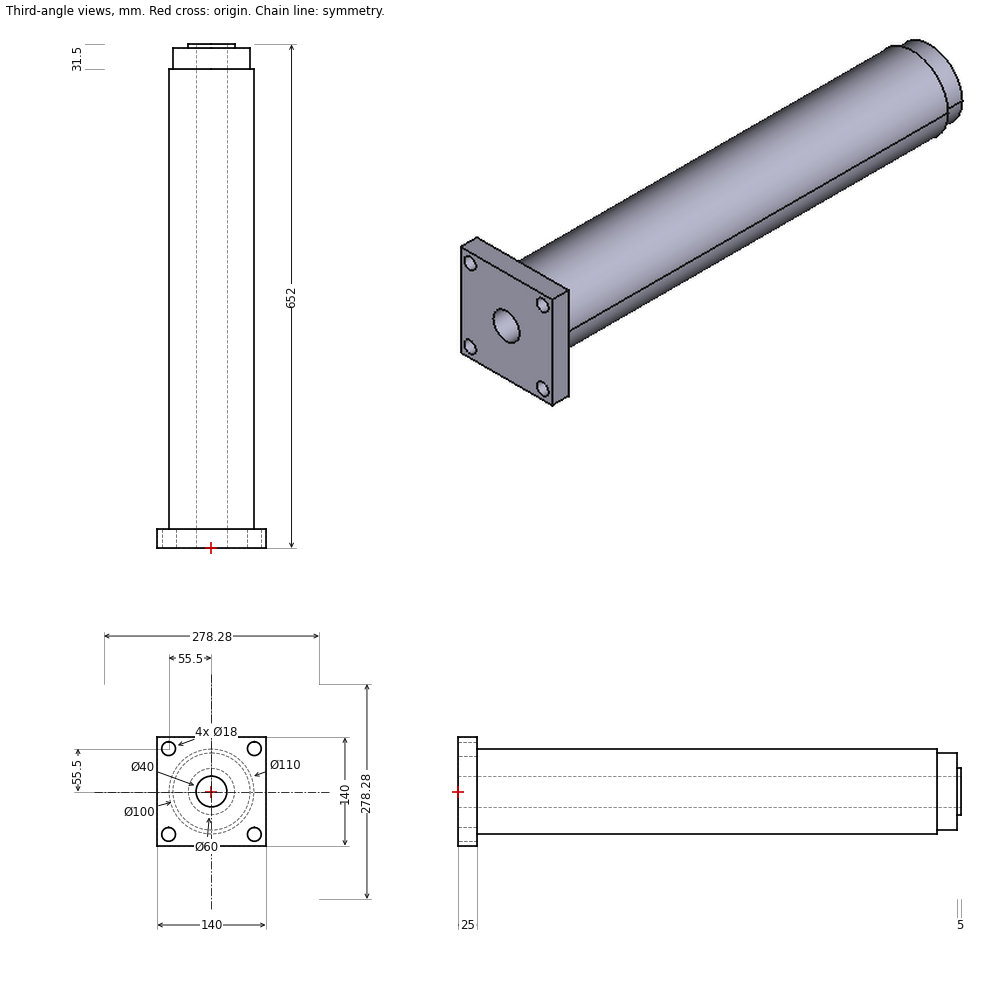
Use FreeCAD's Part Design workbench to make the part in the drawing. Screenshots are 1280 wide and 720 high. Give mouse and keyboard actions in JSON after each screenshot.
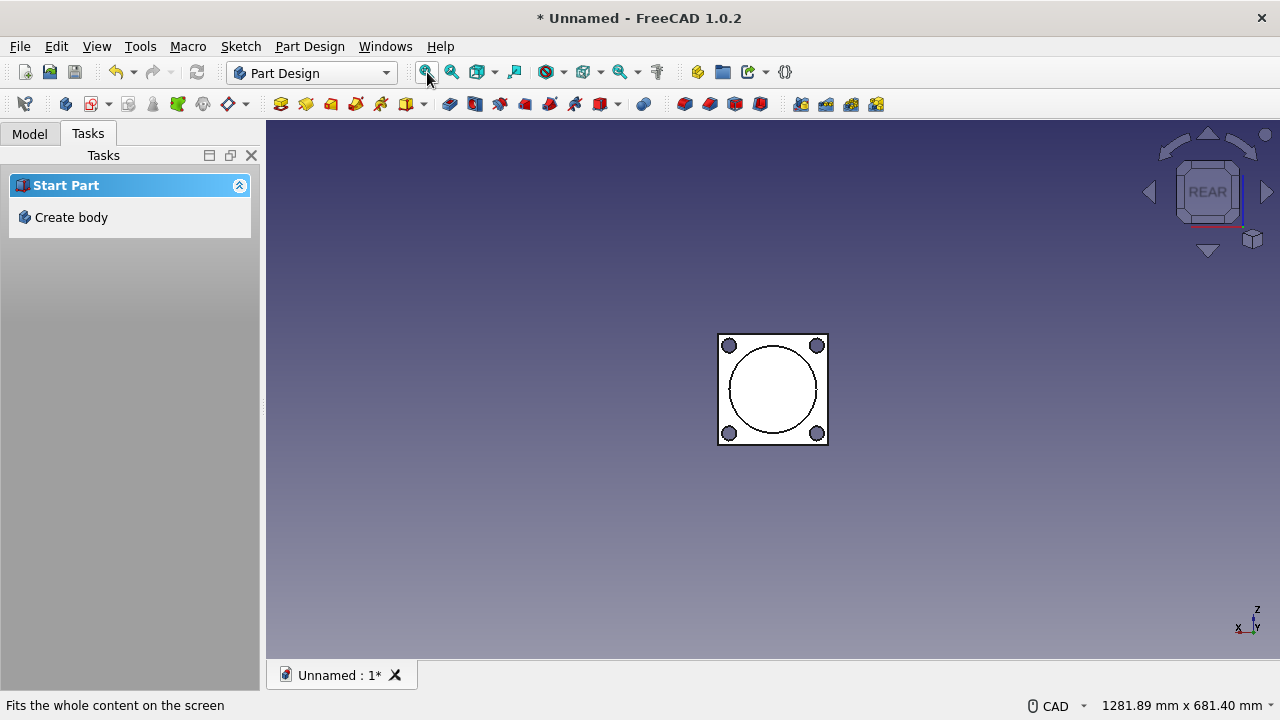
{"action": "left_click", "coordinate": [773, 389]}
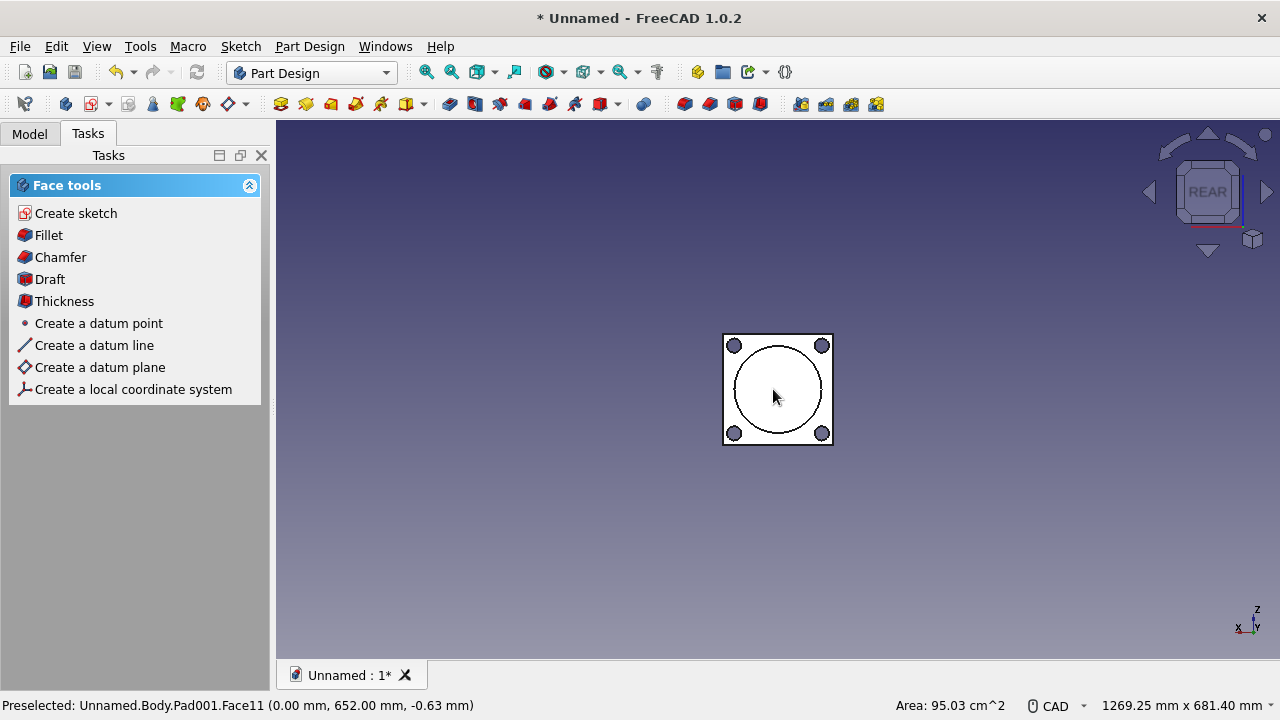
{"action": "left_click", "coordinate": [90, 104]}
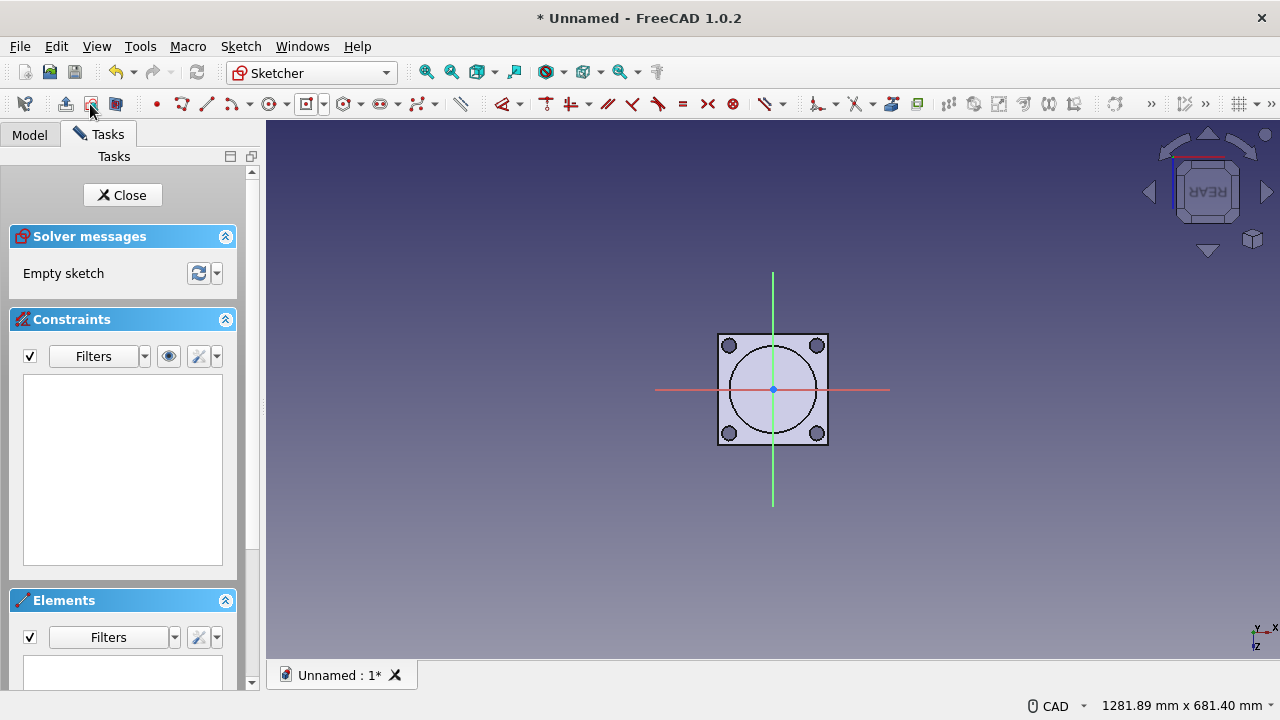
{"action": "scroll", "coordinate": [780, 389], "scroll_direction": "up", "scroll_amount": 12}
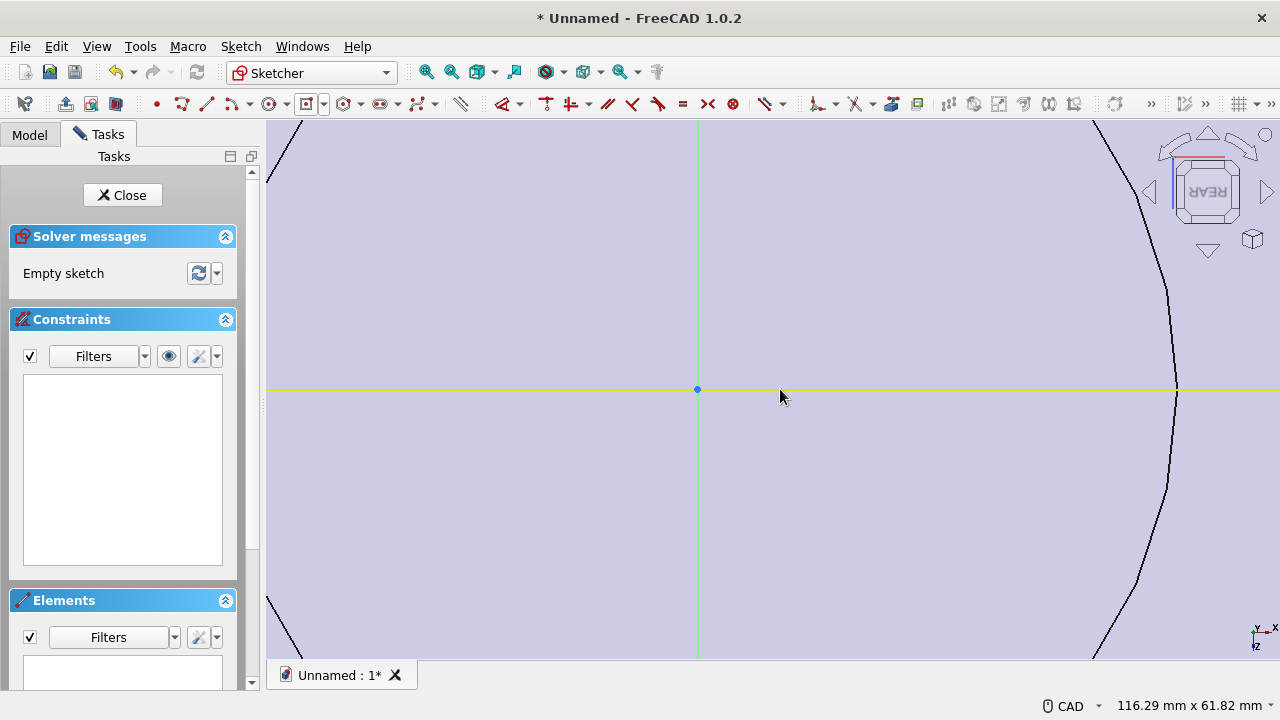
{"action": "key", "text": "g c"}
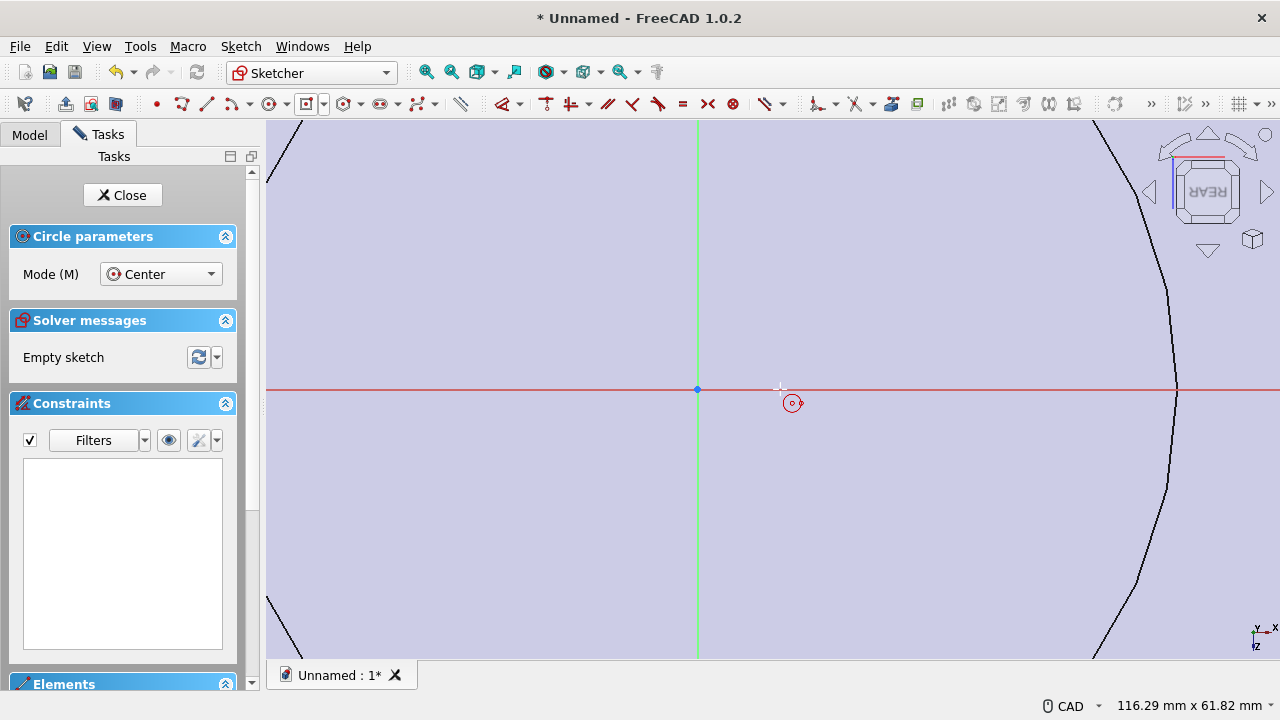
{"action": "left_click", "coordinate": [698, 389]}
{"action": "mouse_move", "coordinate": [821, 266]}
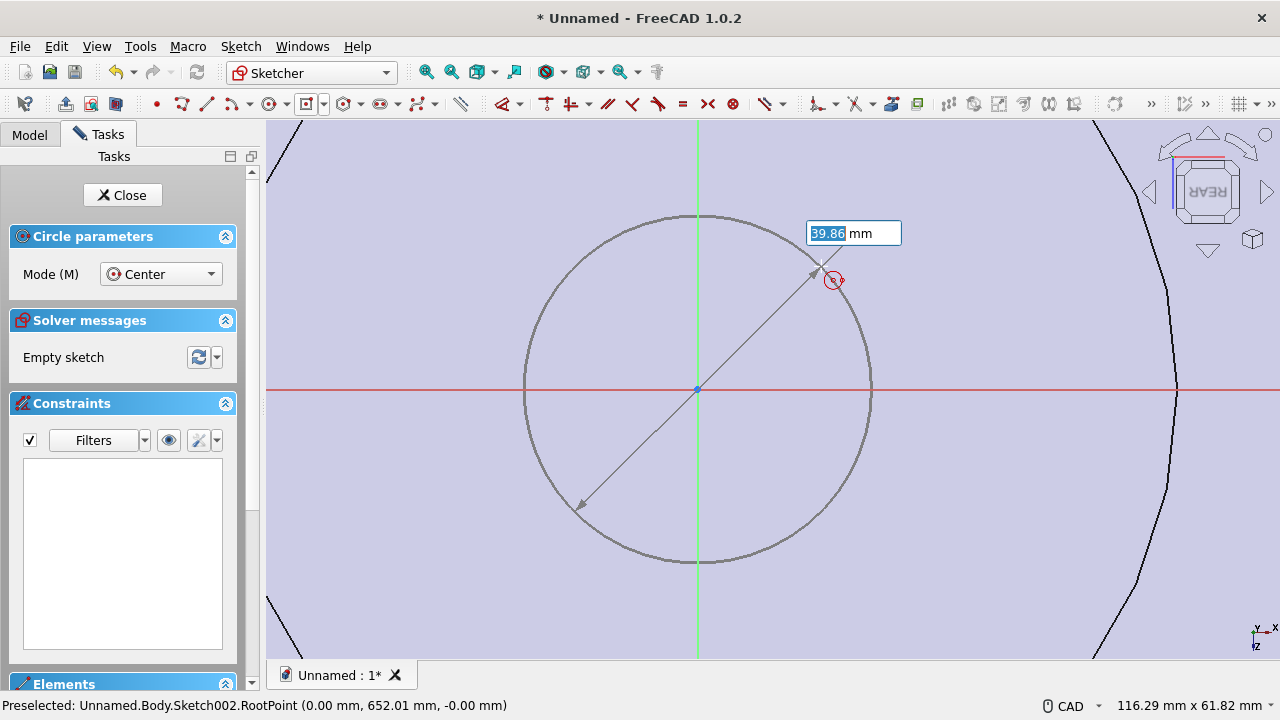
{"action": "type", "text": "40"}
{"action": "key", "text": "Return"}
{"action": "key", "text": "Escape"}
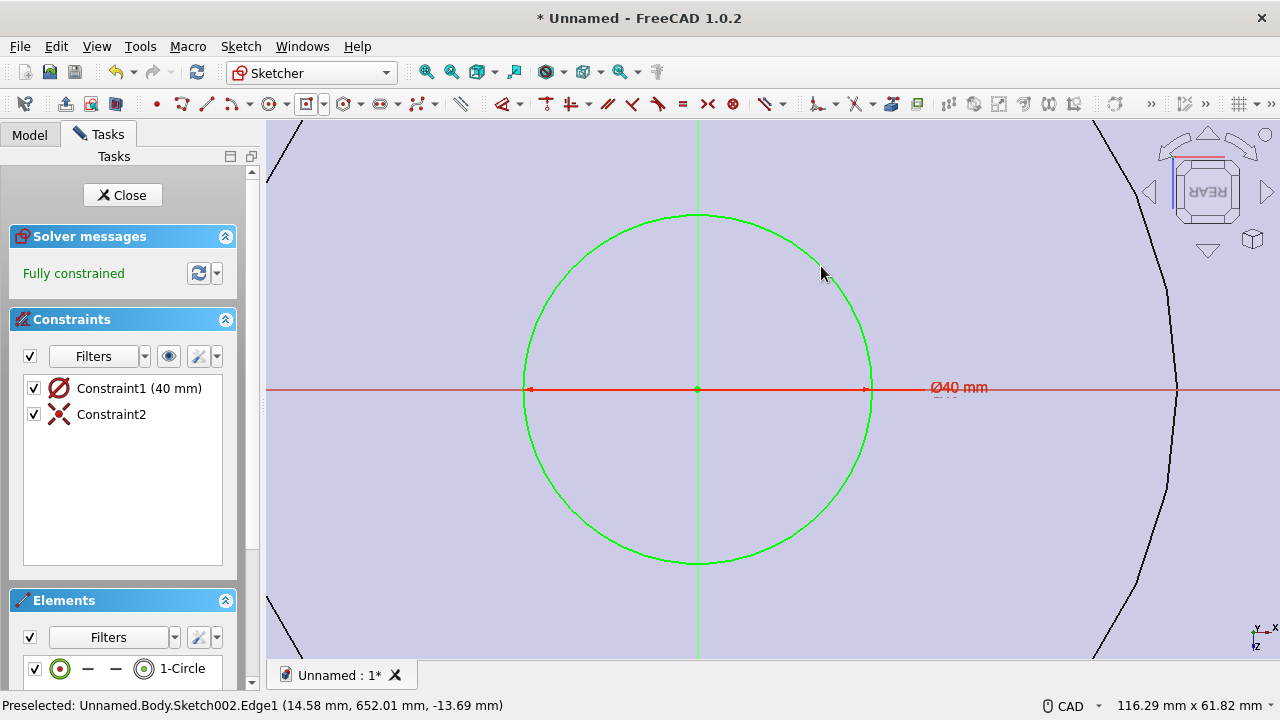
{"action": "left_click", "coordinate": [123, 195]}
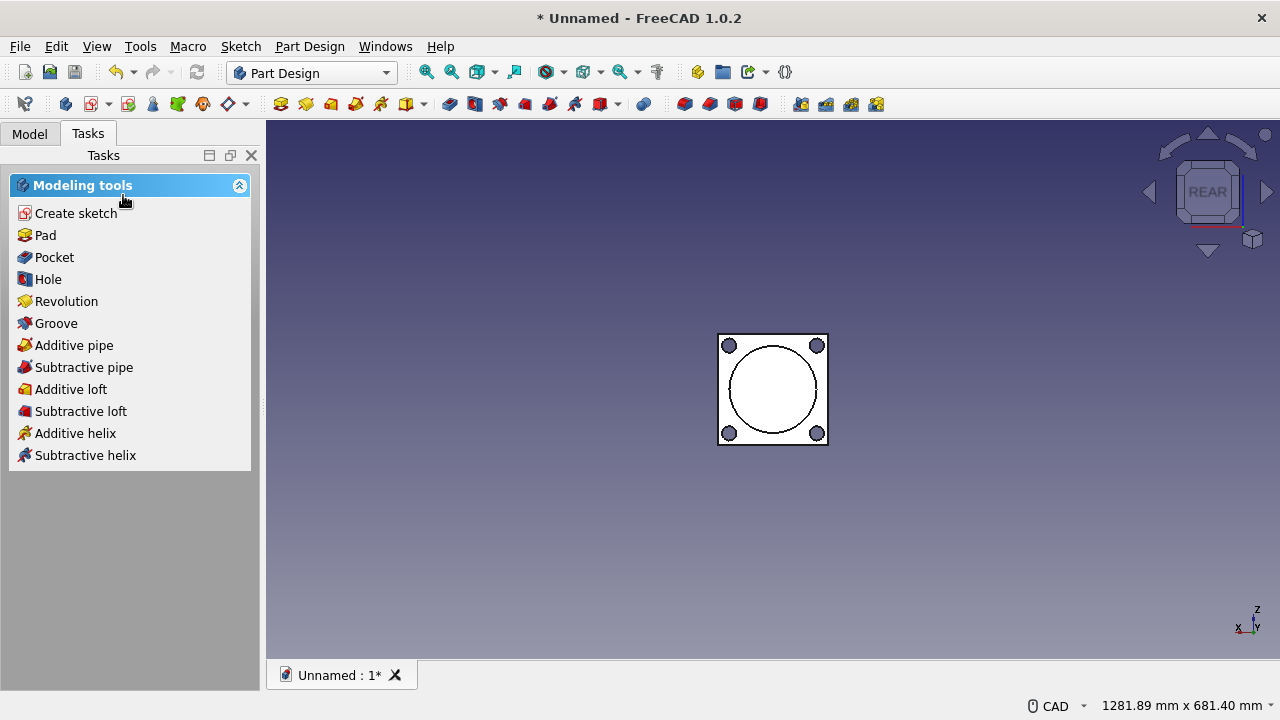
{"action": "left_click", "coordinate": [450, 104]}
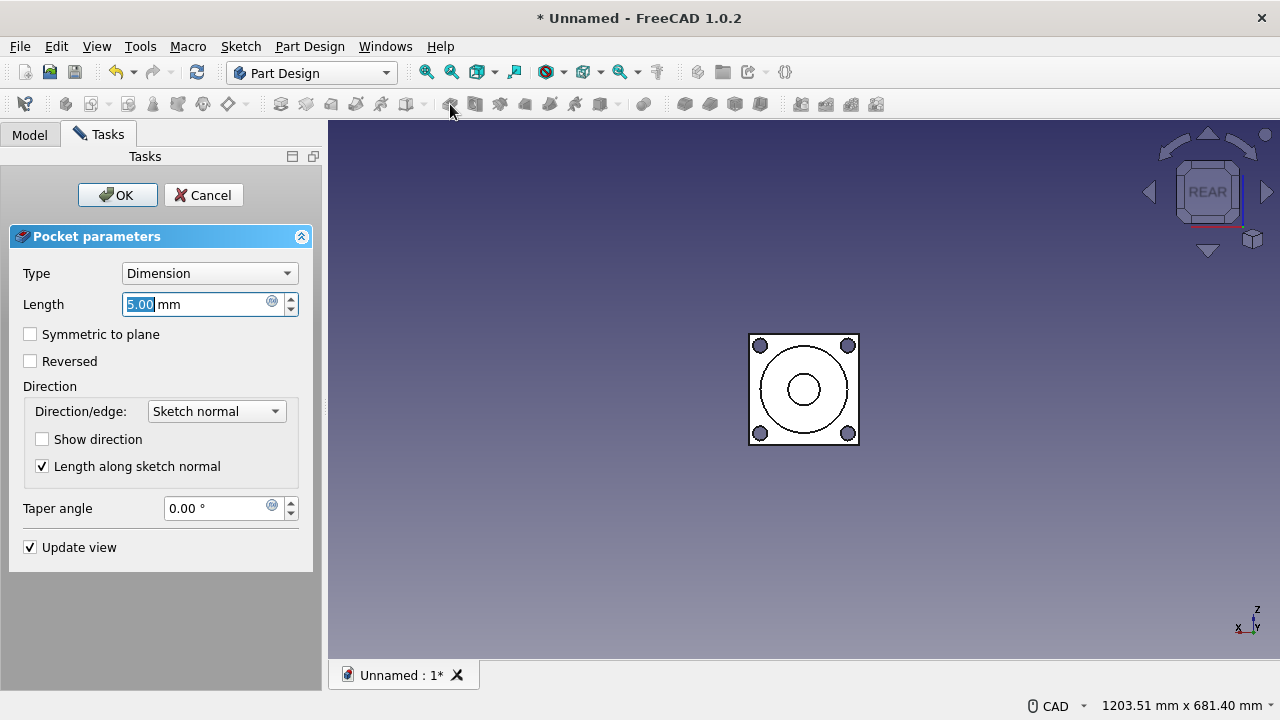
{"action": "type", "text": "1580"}
{"action": "key", "text": "Tab"}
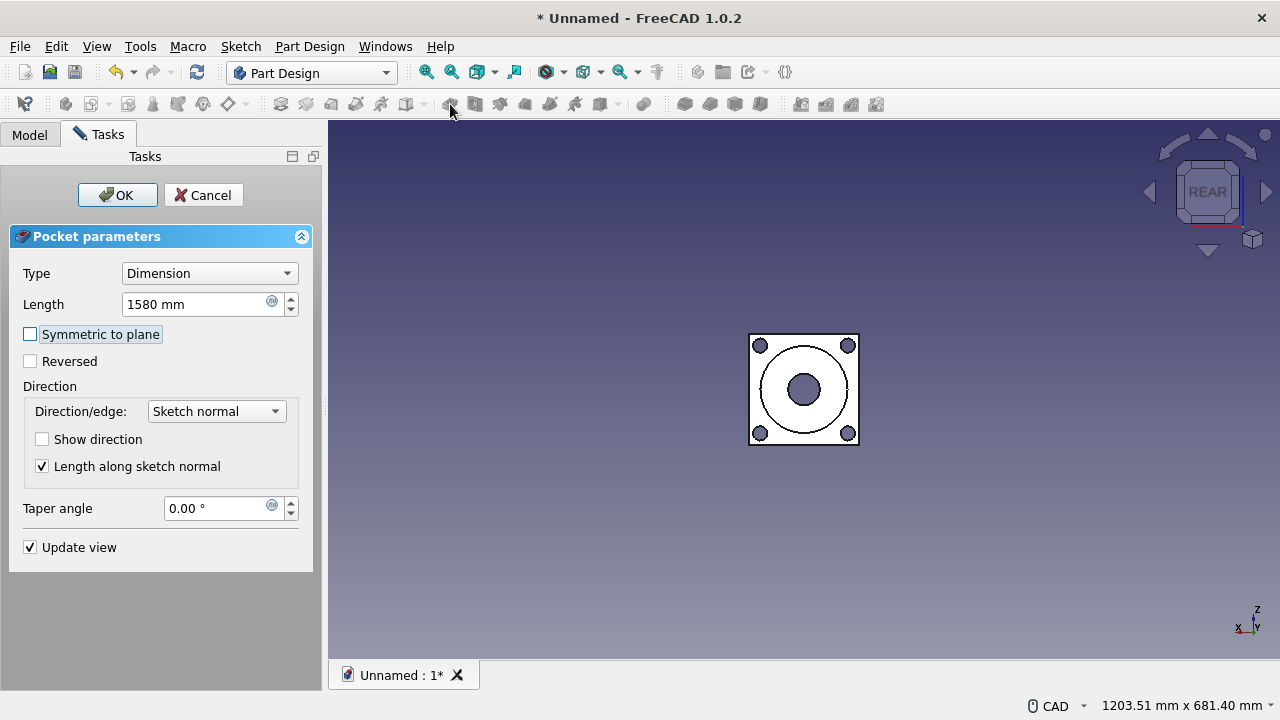
{"action": "left_click", "coordinate": [118, 195]}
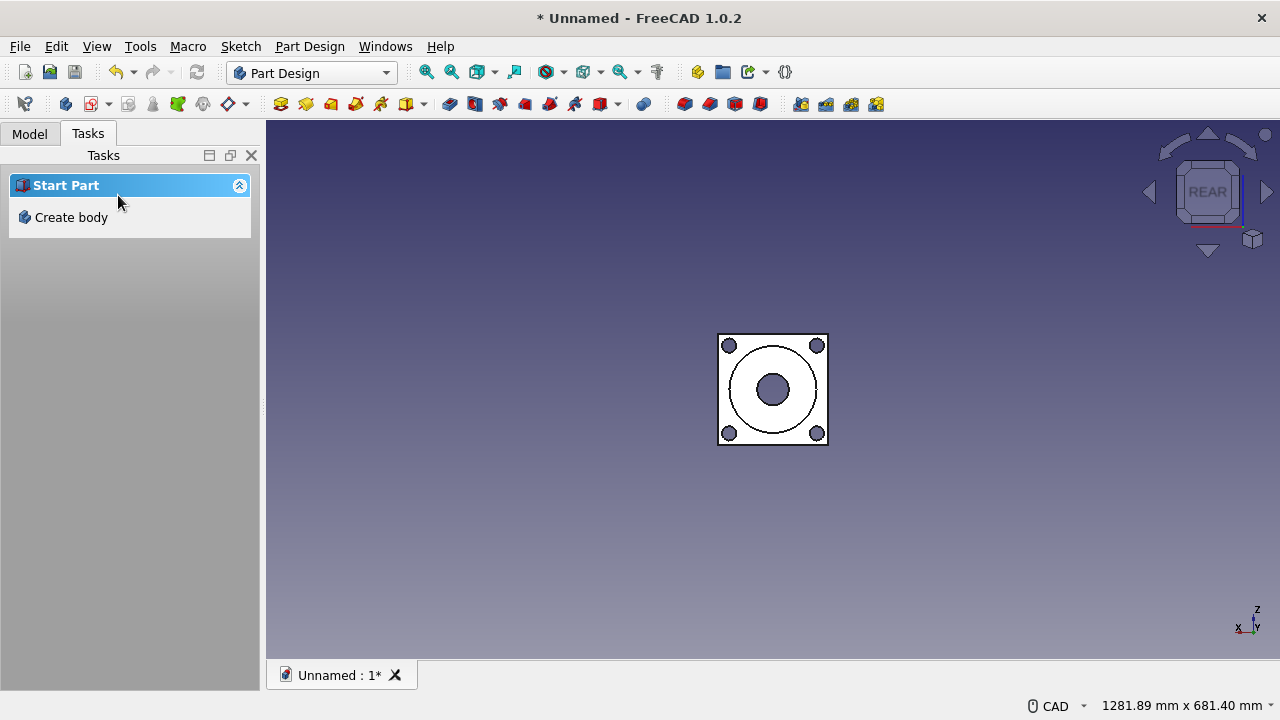
{"action": "key", "text": "v f"}